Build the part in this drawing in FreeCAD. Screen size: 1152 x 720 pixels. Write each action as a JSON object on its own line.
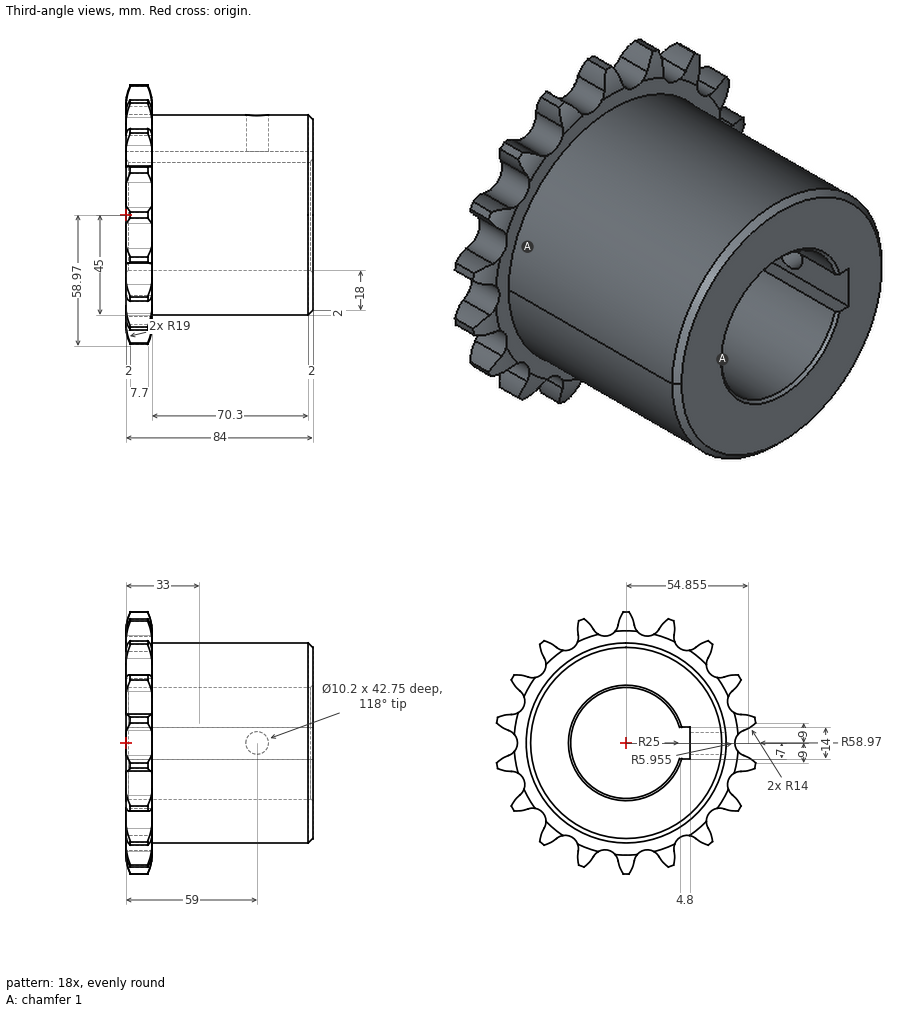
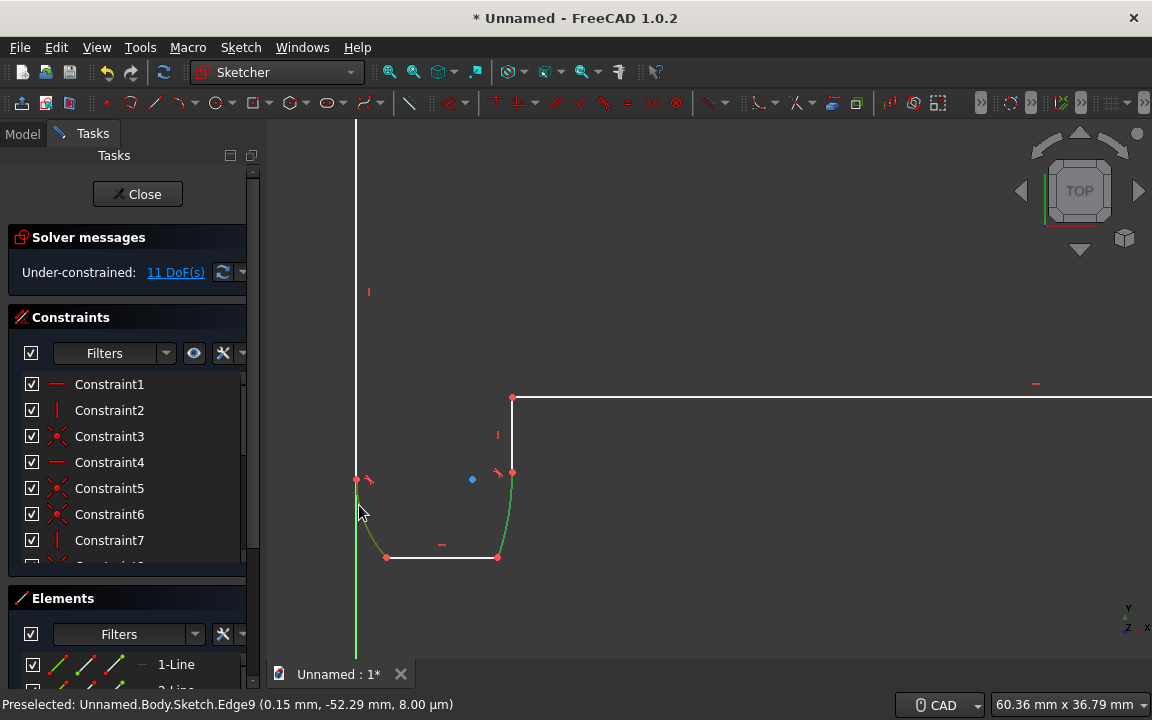
{"action": "key", "text": "e"}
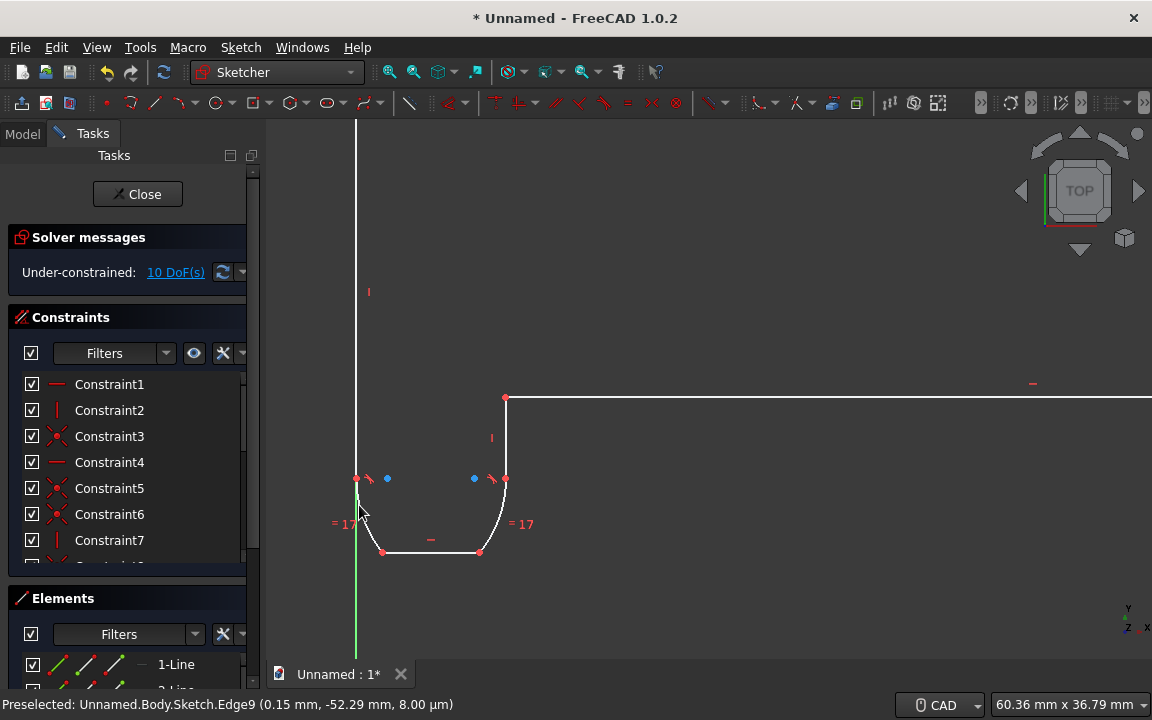
{"action": "key", "text": "d"}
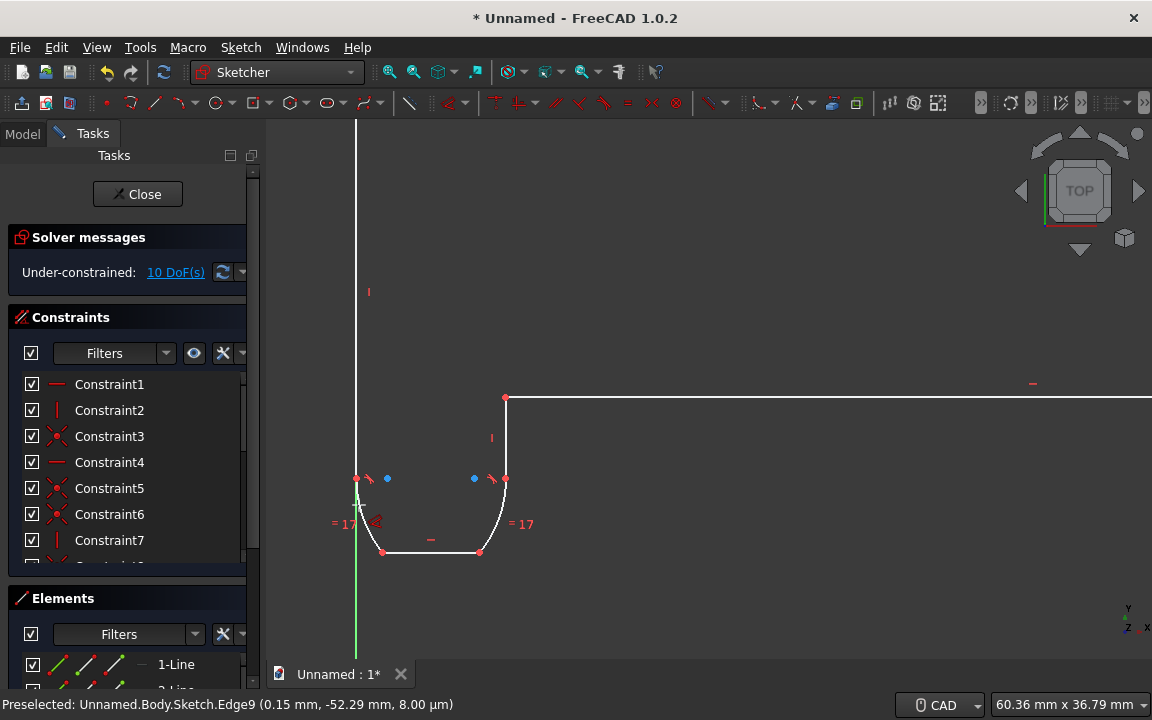
{"action": "left_click", "coordinate": [493, 532]}
{"action": "left_click", "coordinate": [522, 547]}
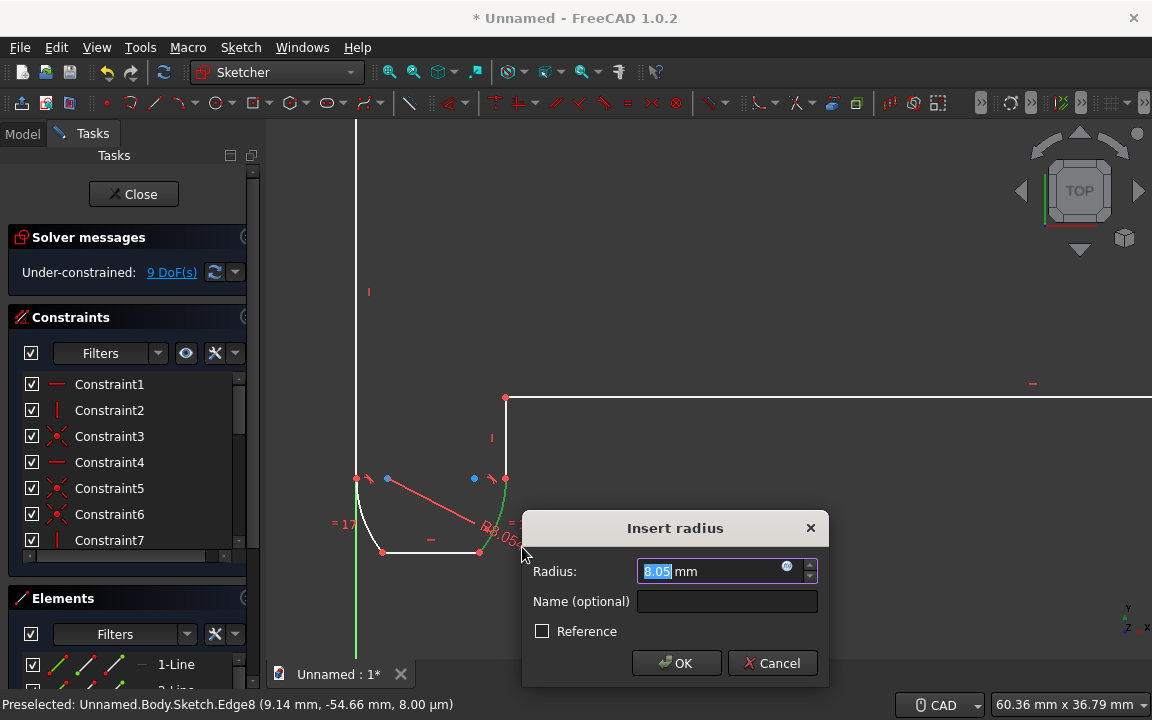
{"action": "type", "text": "19"}
{"action": "key", "text": "Return"}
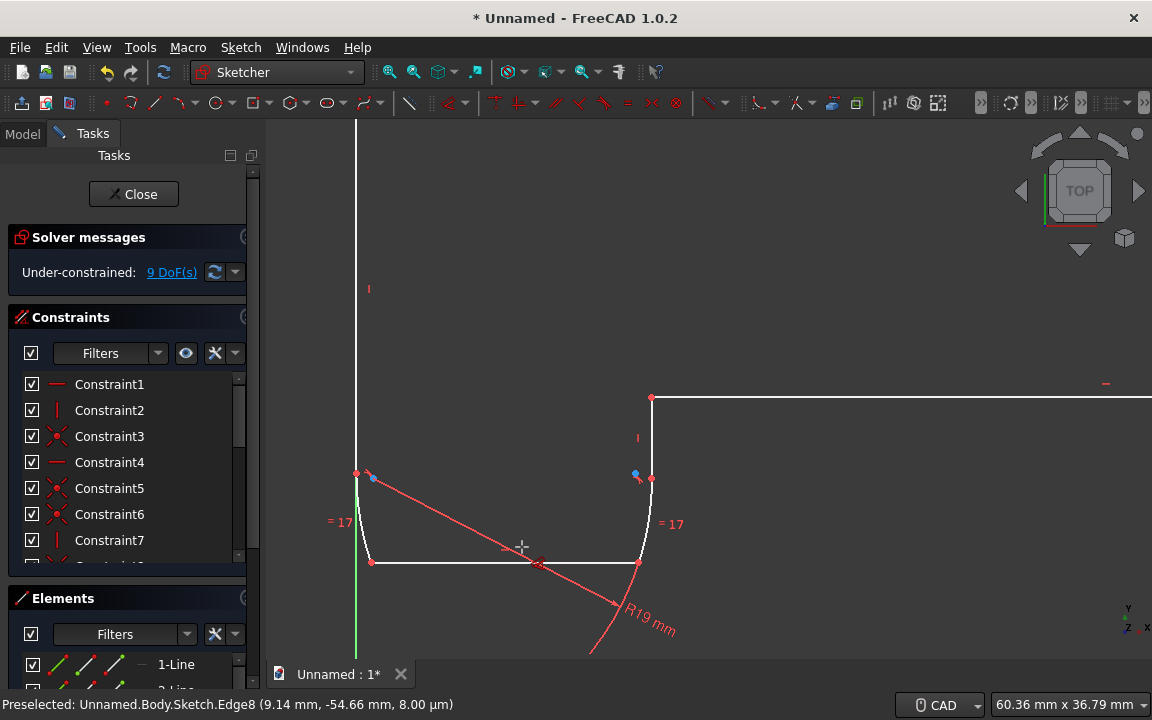
{"action": "scroll", "coordinate": [447, 518], "scroll_direction": "down", "scroll_amount": 5}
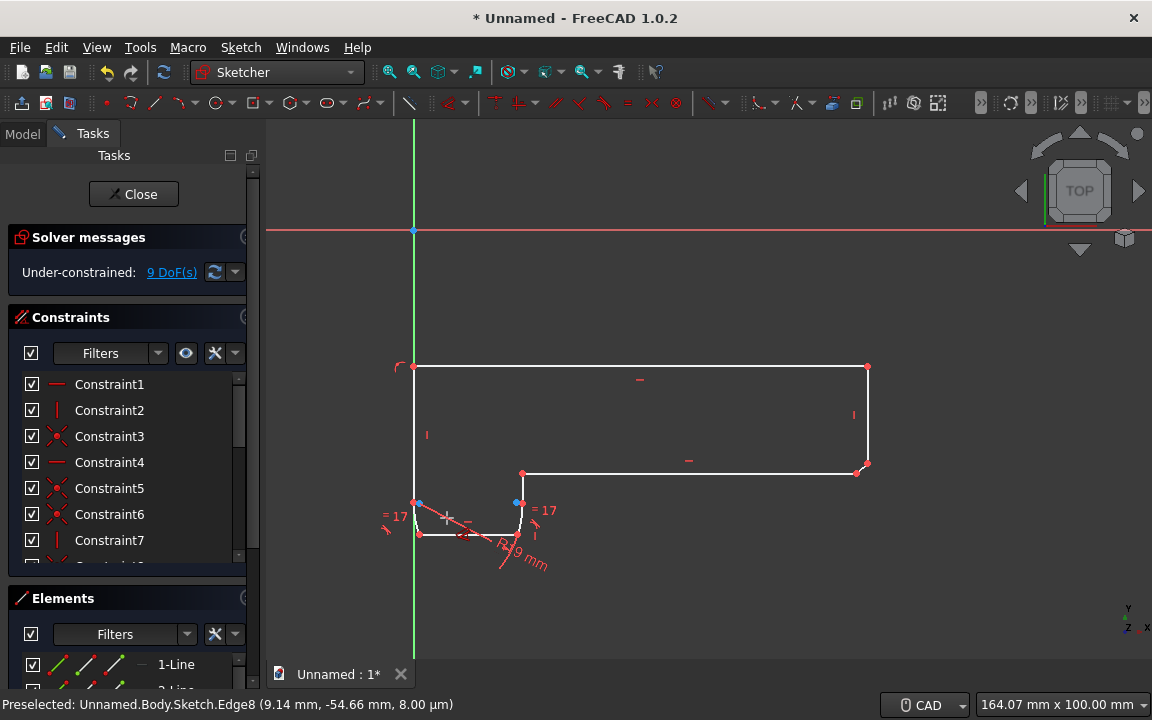
{"action": "left_click", "coordinate": [868, 434]}
{"action": "left_click", "coordinate": [902, 415]}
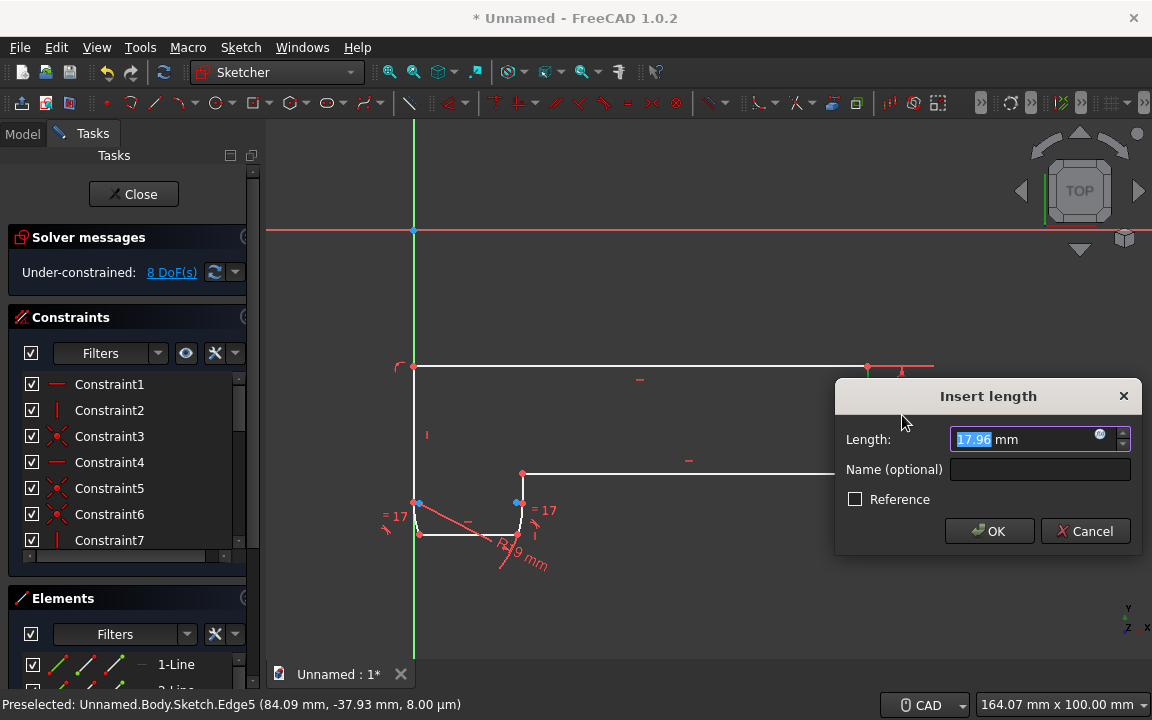
{"action": "type", "text": "18"}
{"action": "key", "text": "Return"}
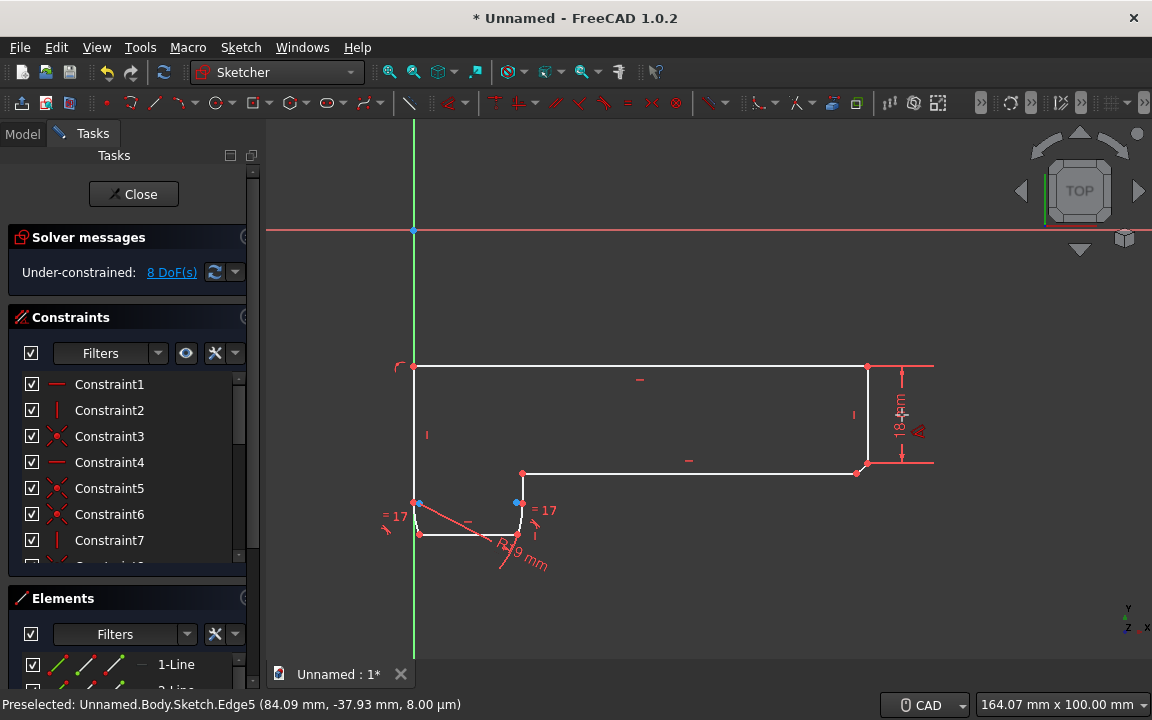
{"action": "left_click", "coordinate": [732, 366]}
{"action": "left_click", "coordinate": [641, 332]}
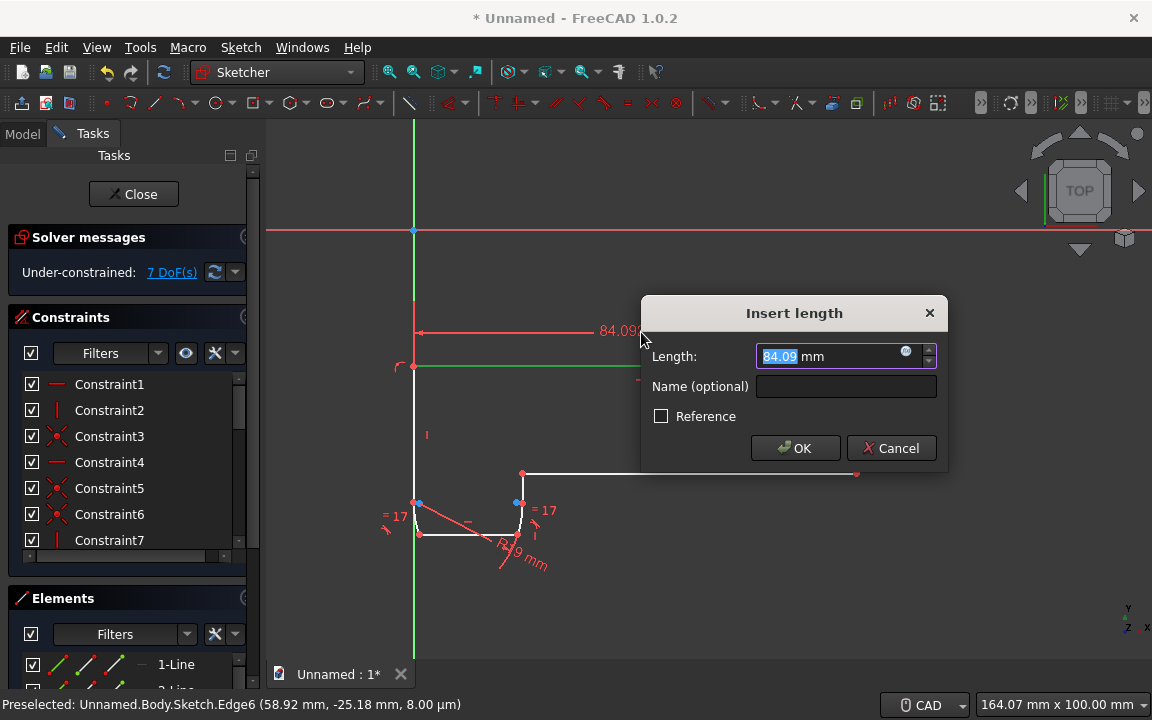
{"action": "type", "text": "84"}
{"action": "key", "text": "Return"}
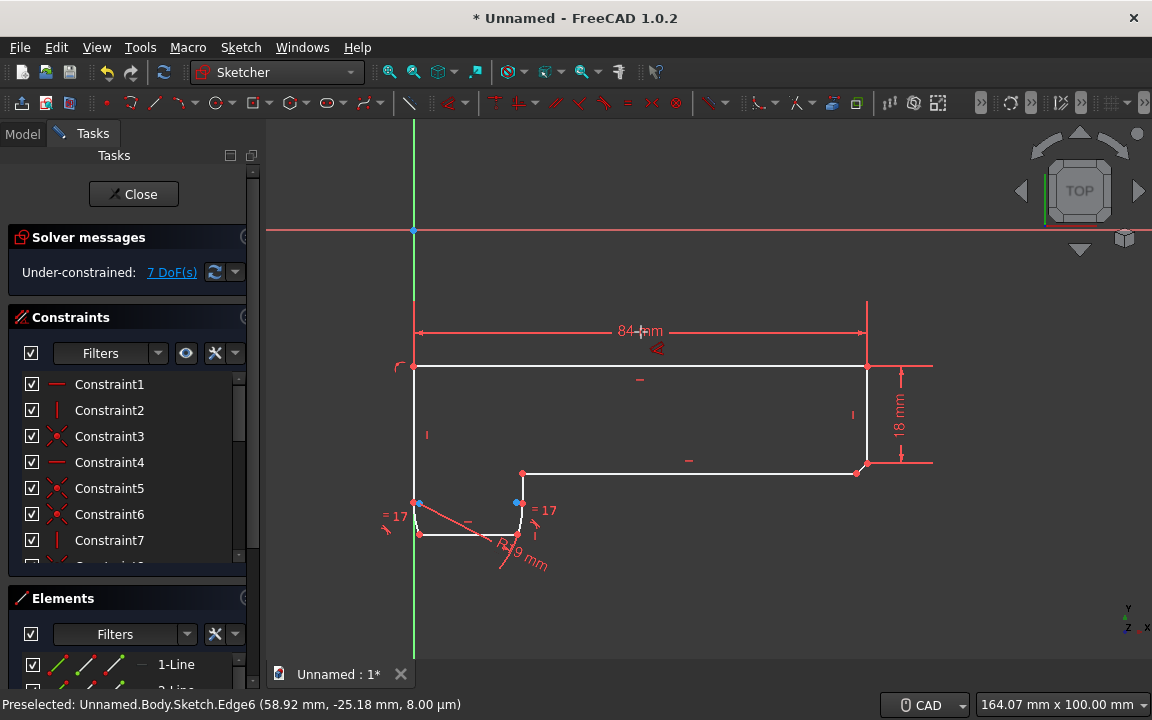
{"action": "scroll", "coordinate": [419, 535], "scroll_direction": "up", "scroll_amount": 7}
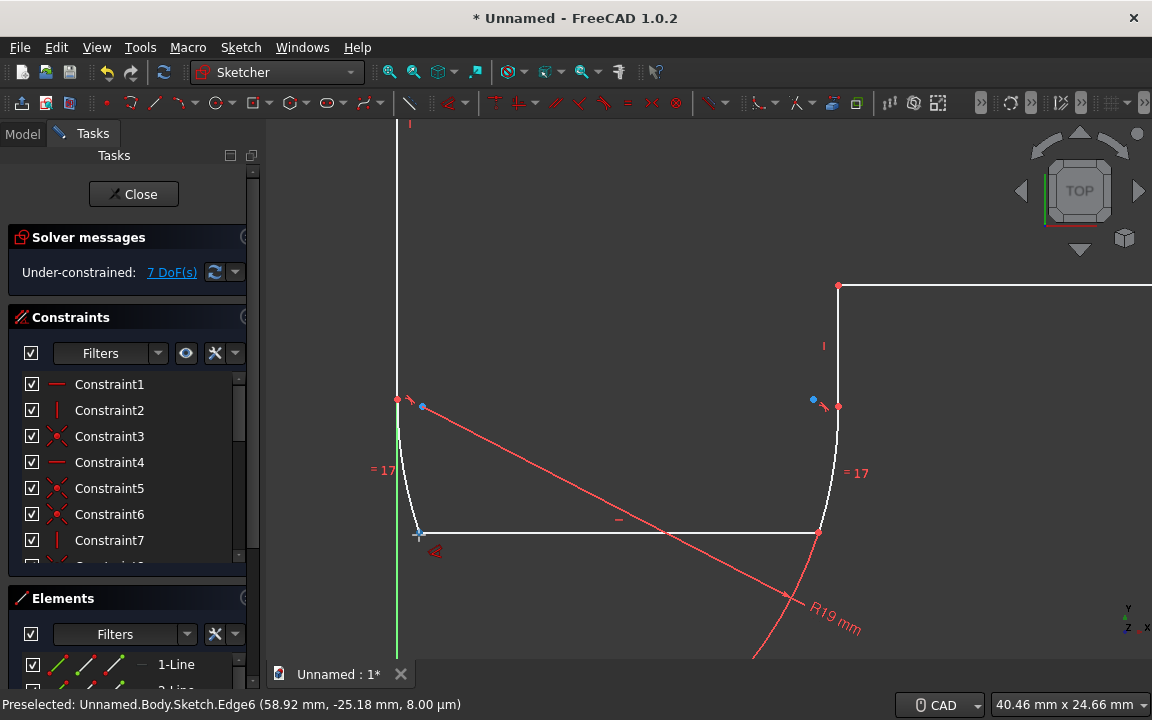
{"action": "left_click", "coordinate": [419, 533]}
{"action": "left_click", "coordinate": [414, 567]}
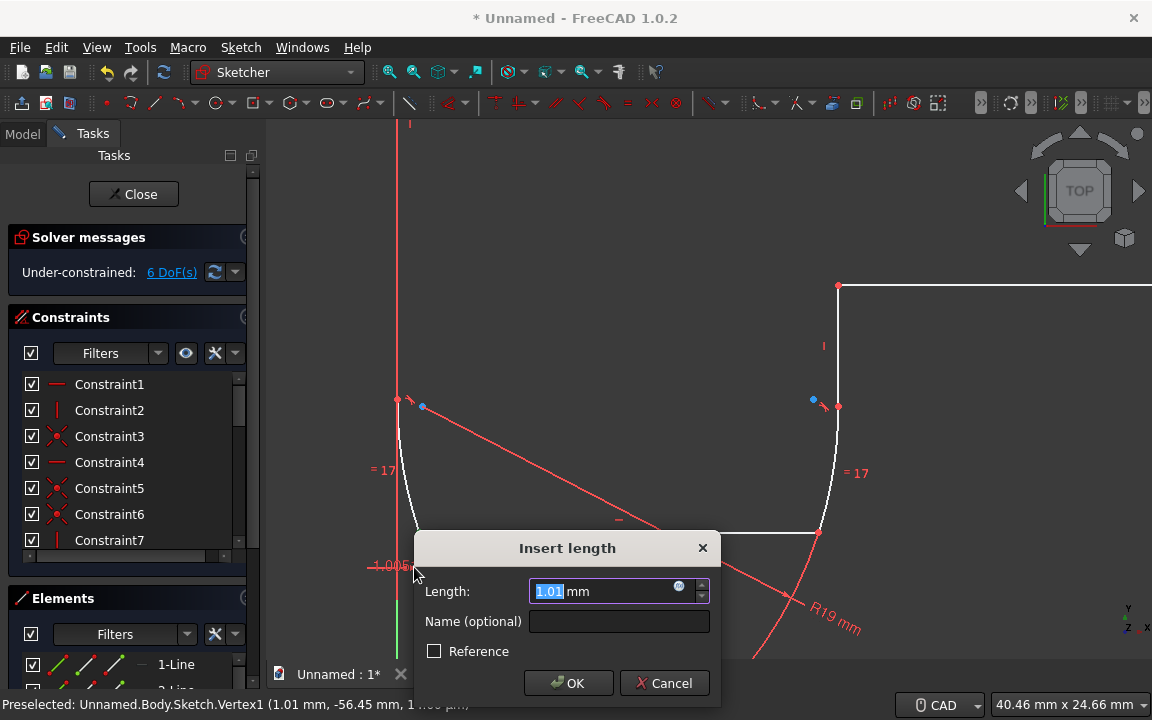
{"action": "type", "text": "2"}
{"action": "key", "text": "Return"}